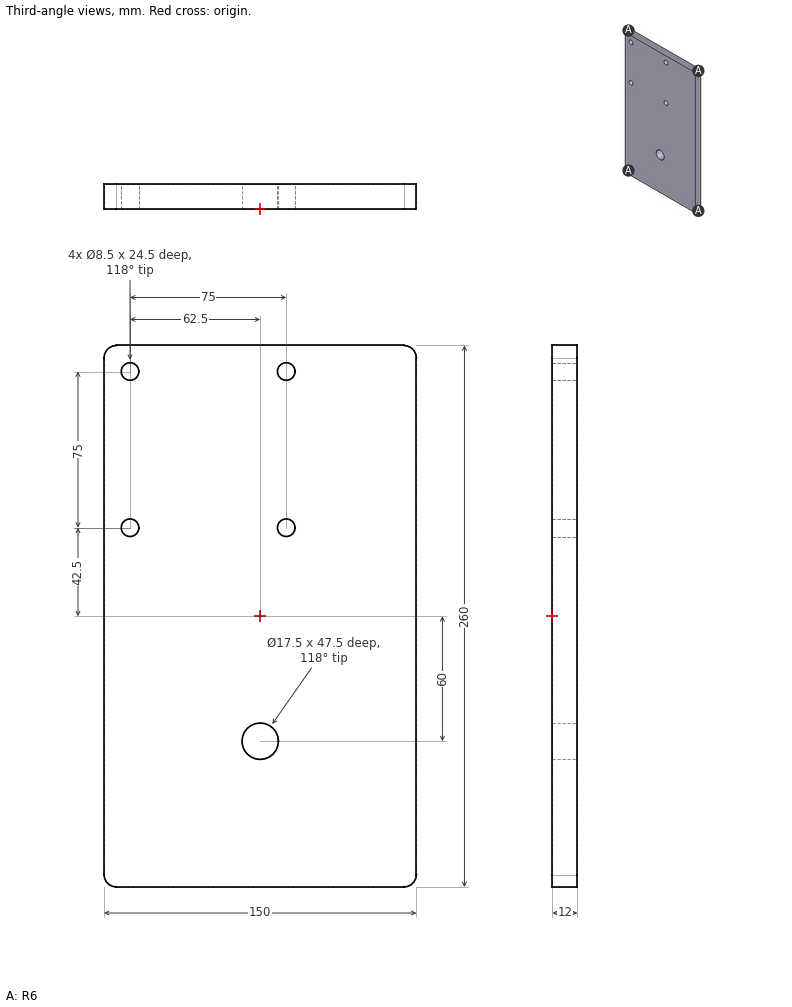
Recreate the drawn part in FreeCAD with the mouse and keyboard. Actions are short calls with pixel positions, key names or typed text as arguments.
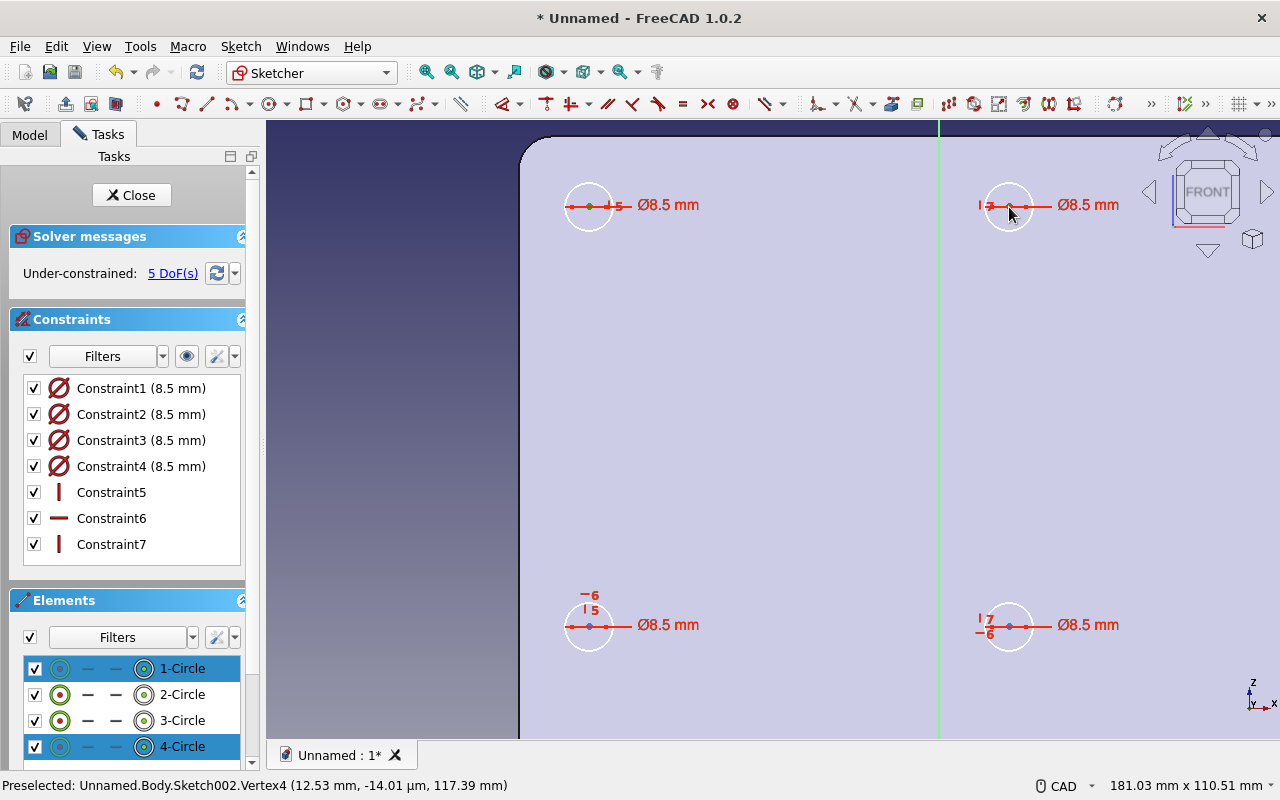
key(h)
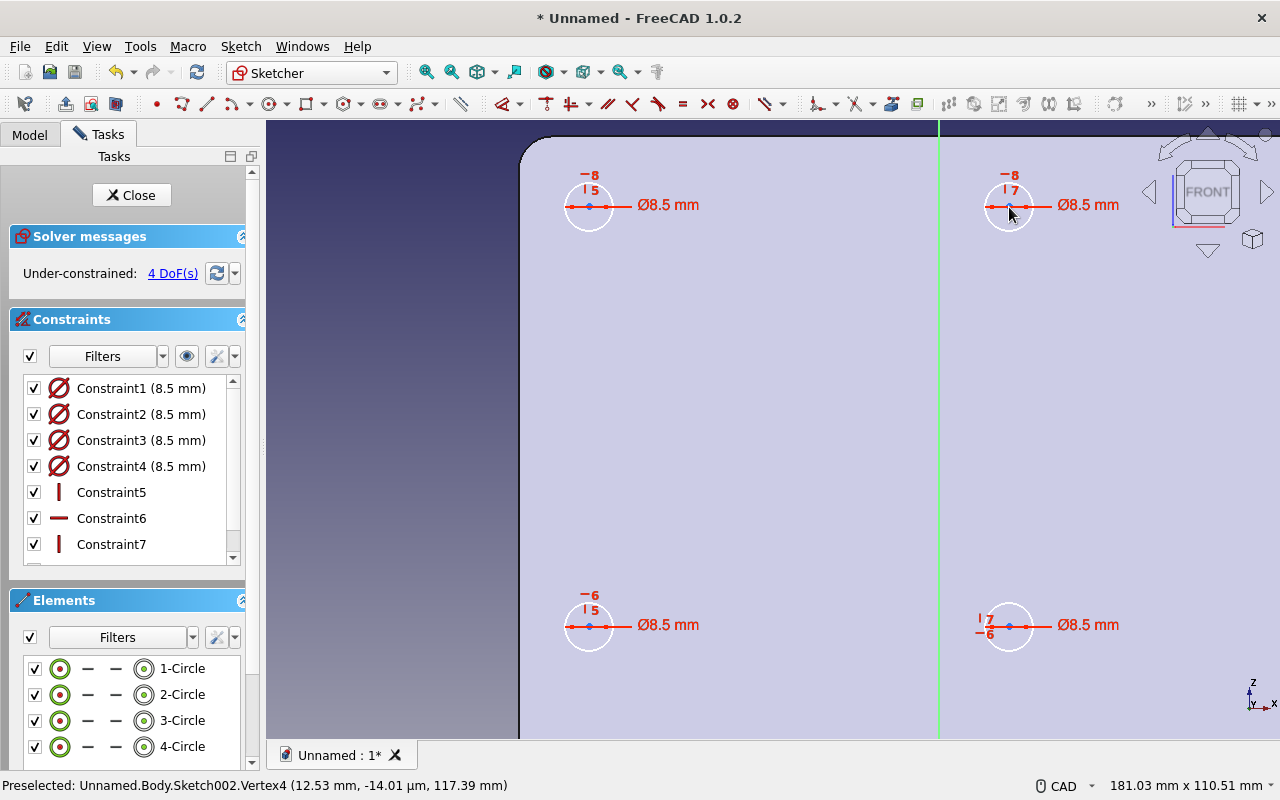
click(502, 104)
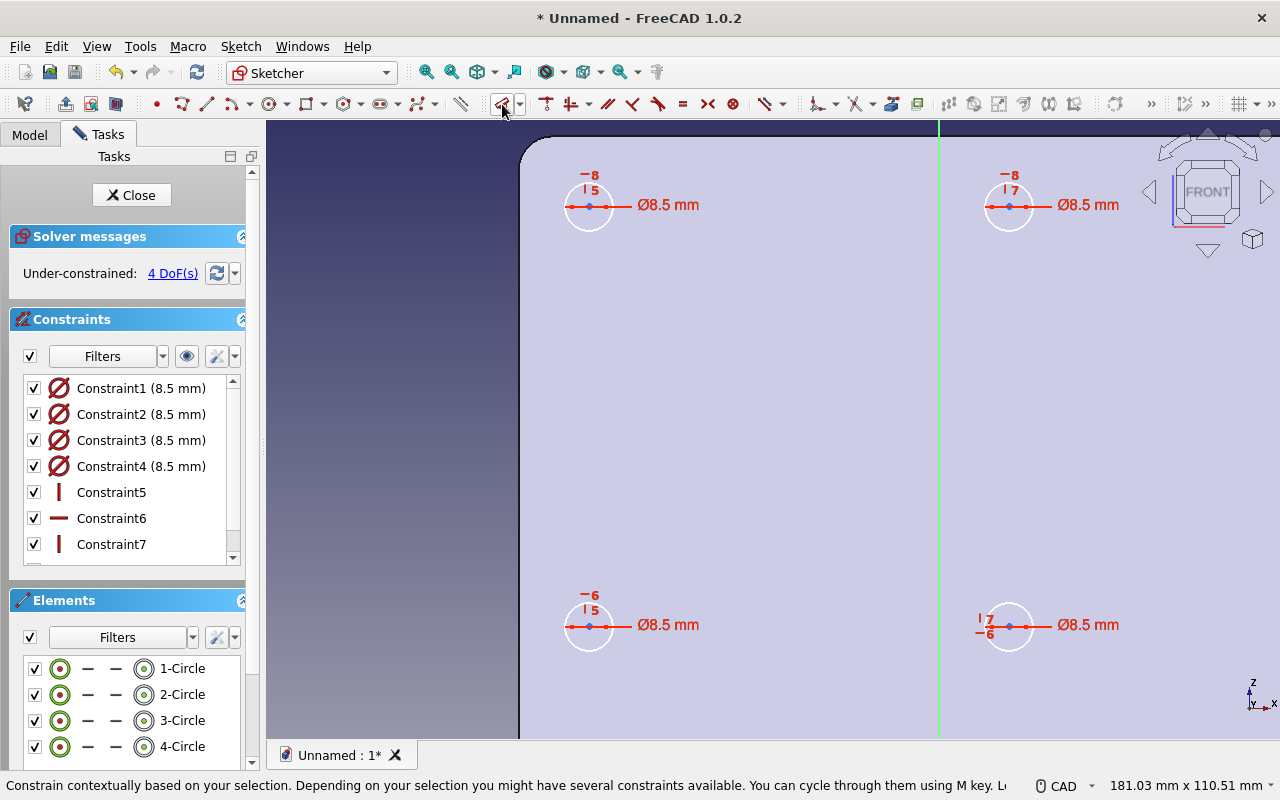
click(589, 207)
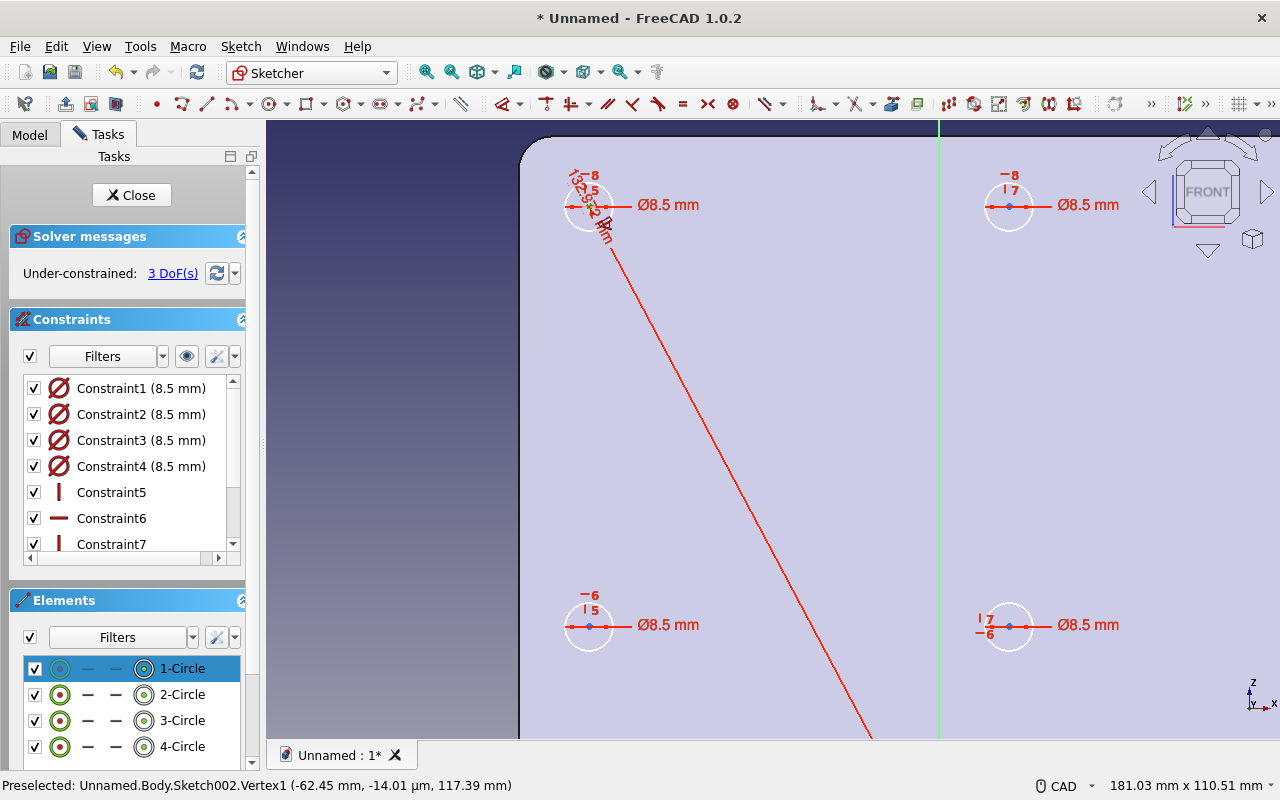
click(589, 627)
click(555, 417)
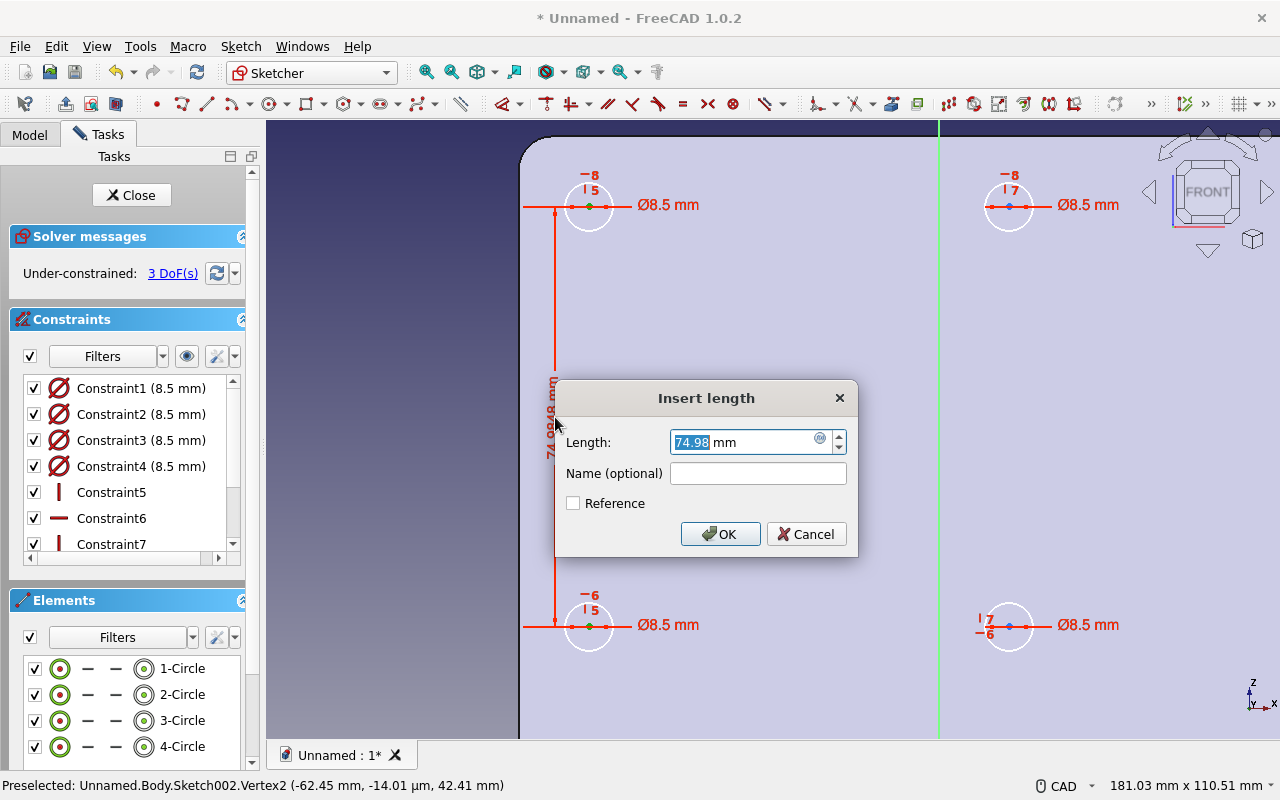
text(75)
key(Return)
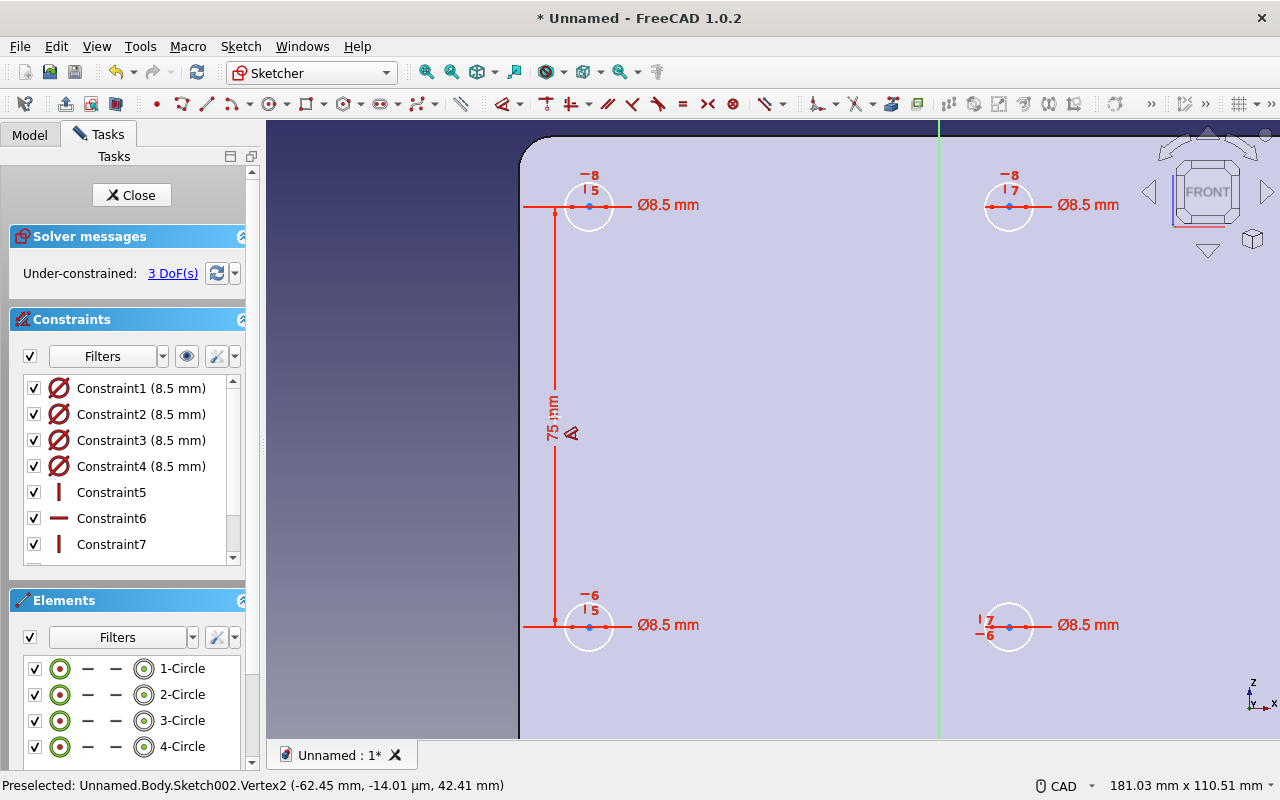
click(589, 627)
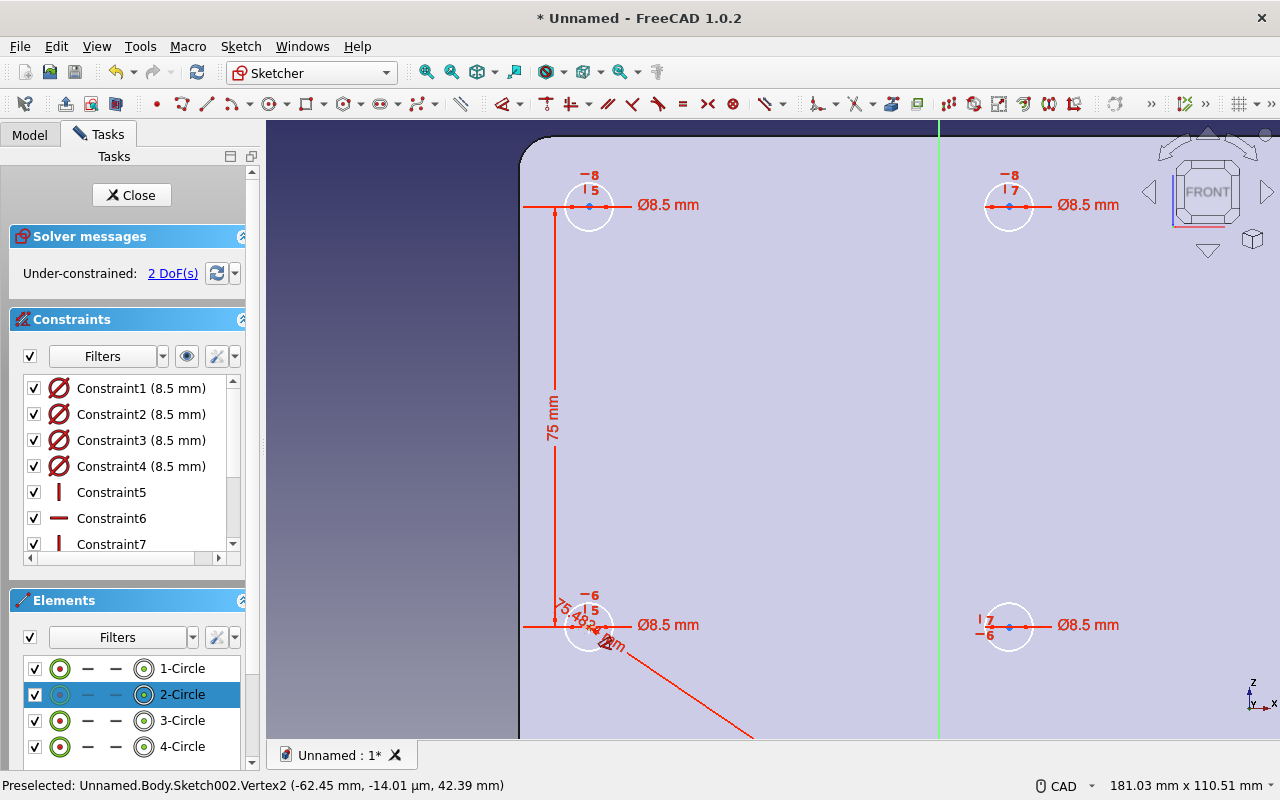
click(1009, 627)
click(799, 661)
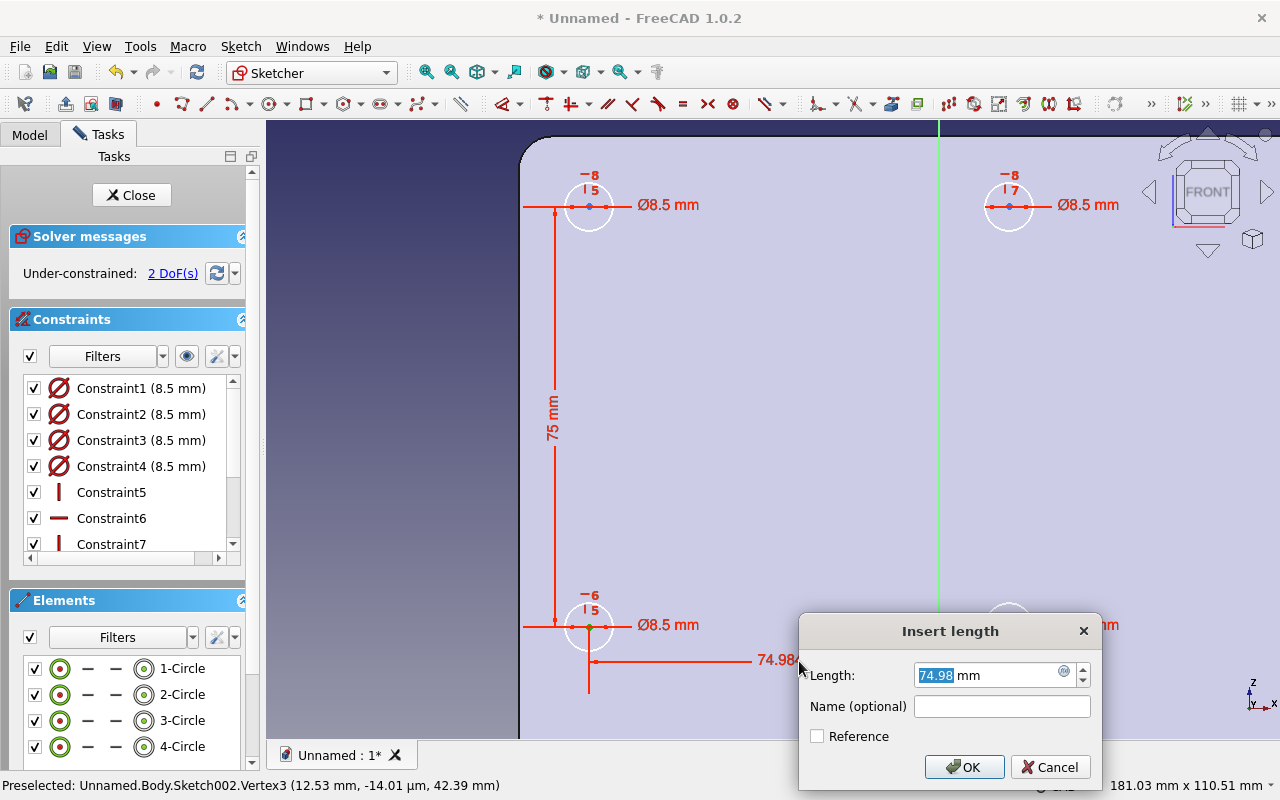
text(75)
key(Return)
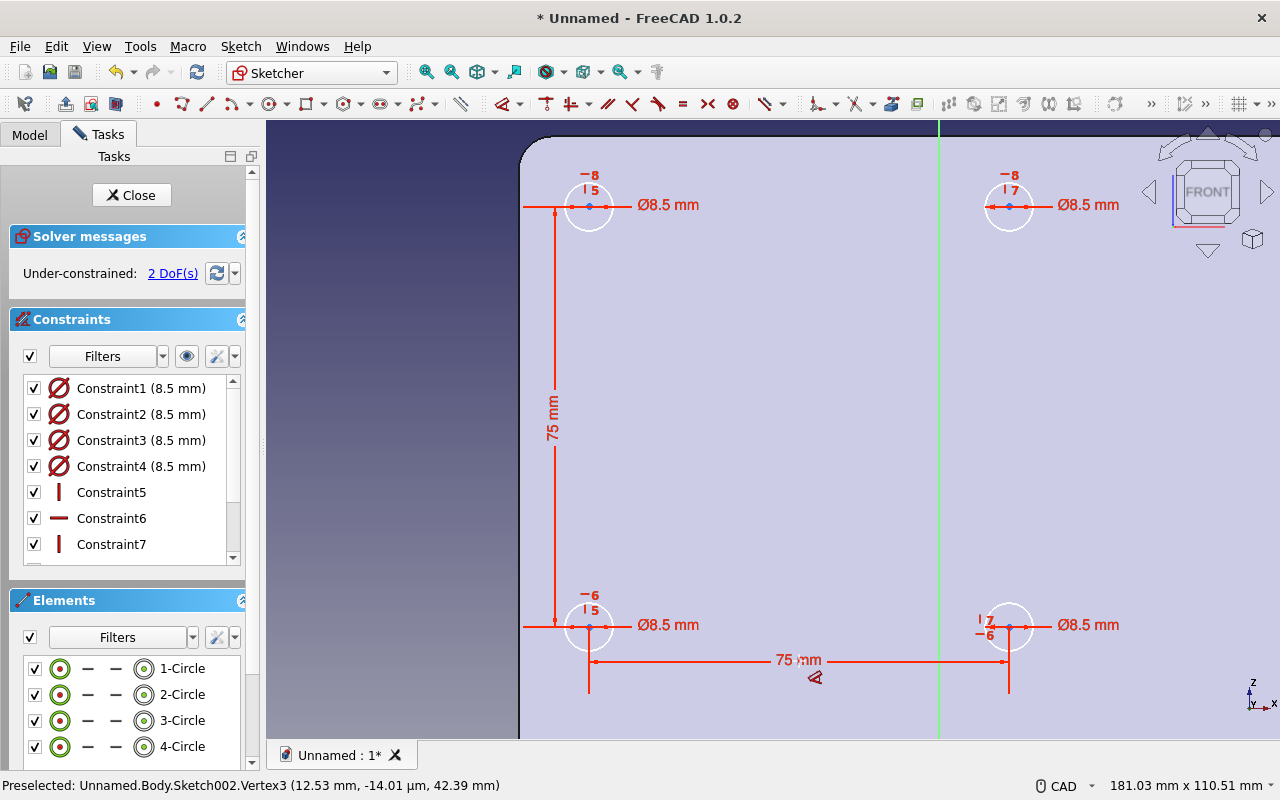
click(589, 207)
click(764, 173)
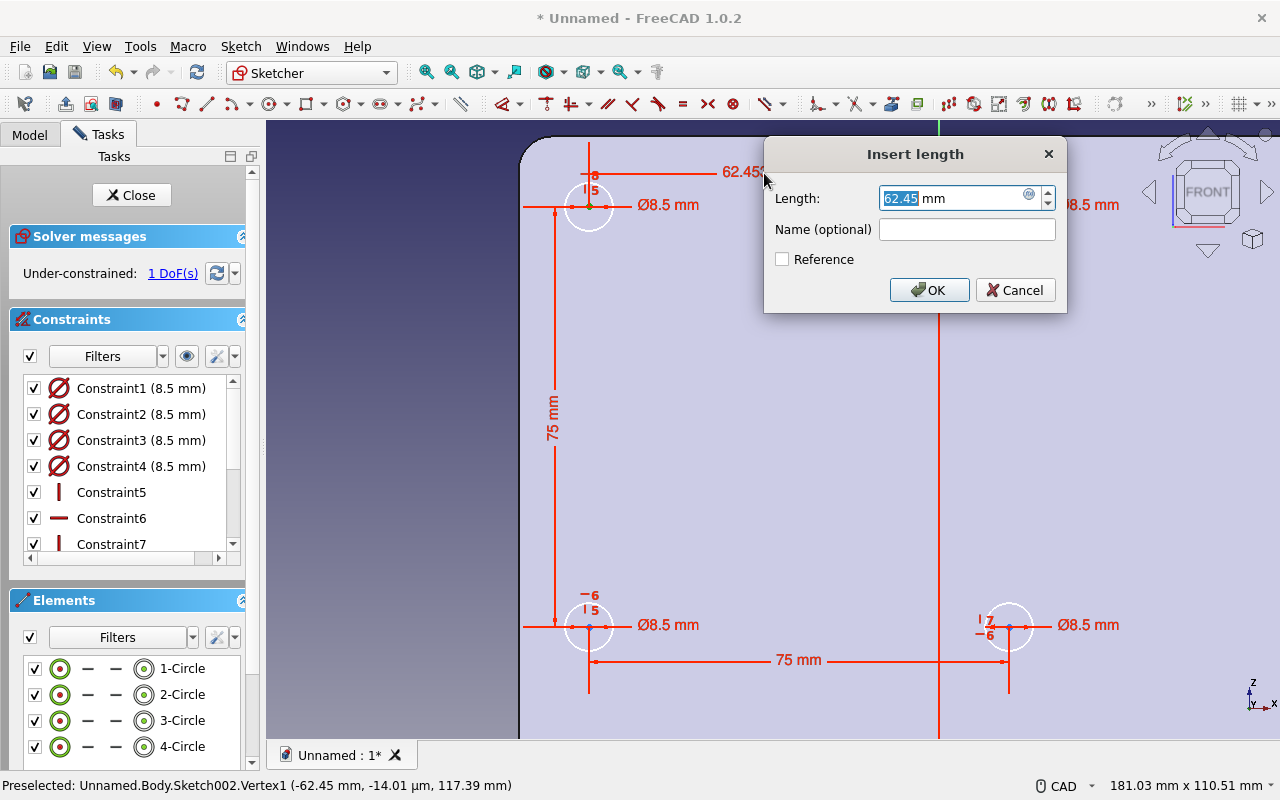
text(62.5)
key(Return)